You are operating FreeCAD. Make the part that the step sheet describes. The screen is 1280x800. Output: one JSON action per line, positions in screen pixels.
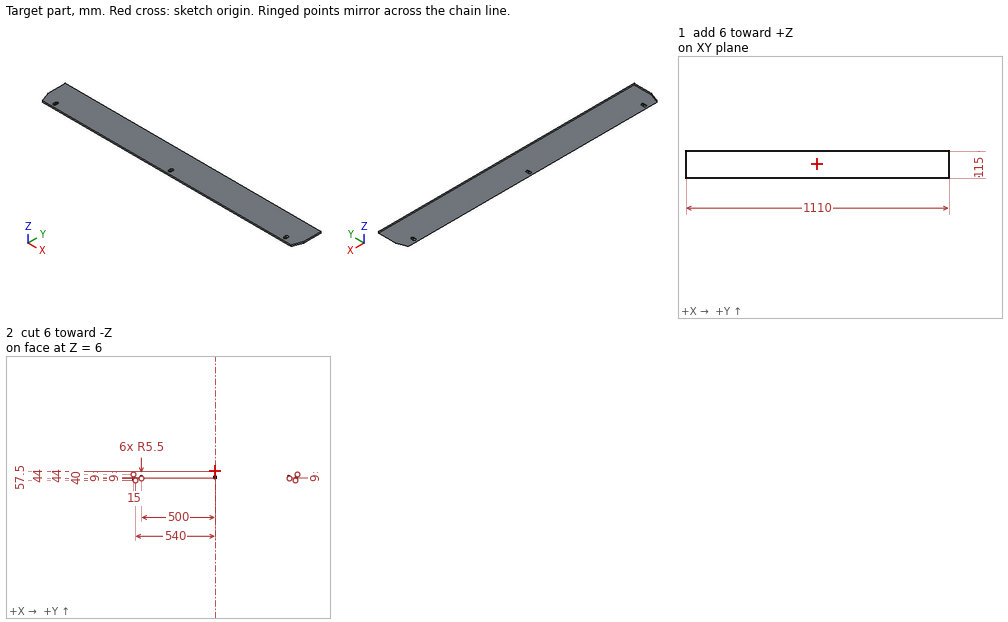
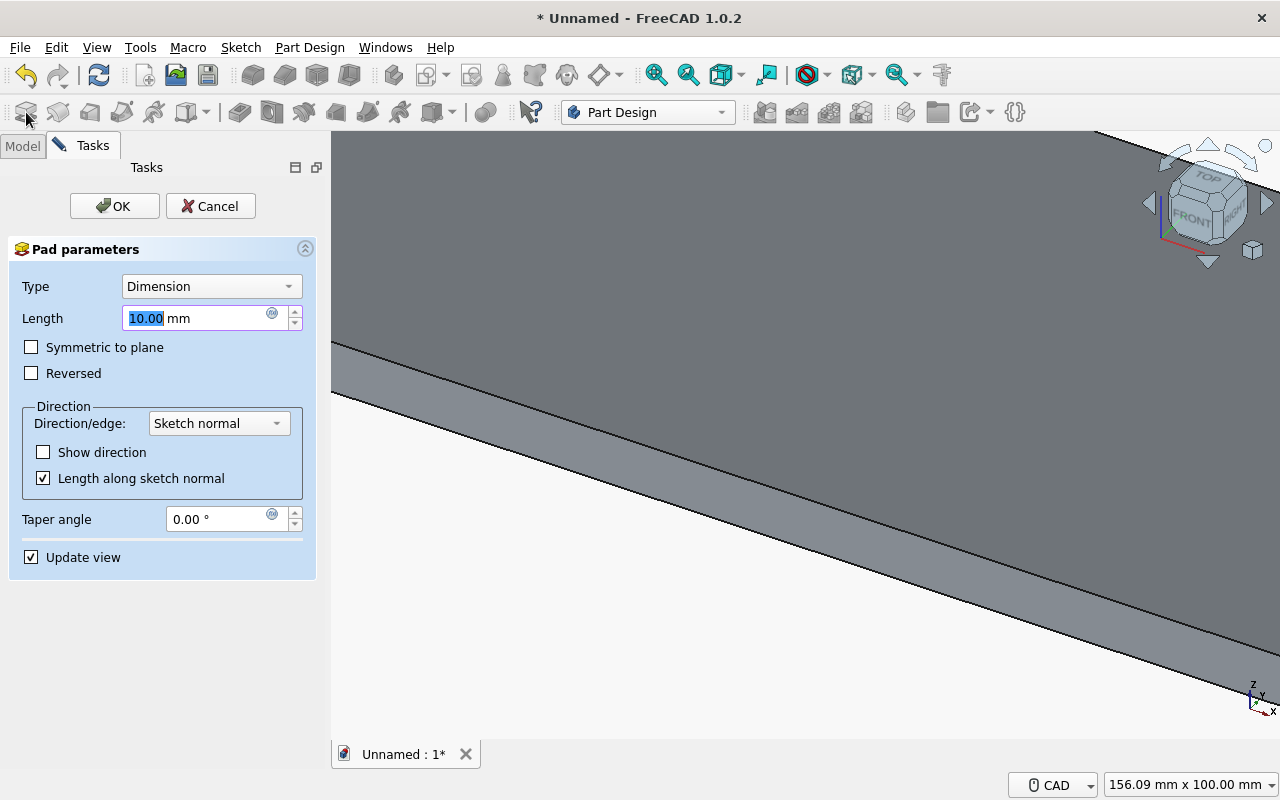
{"action": "type", "text": "6"}
{"action": "key", "text": "Tab"}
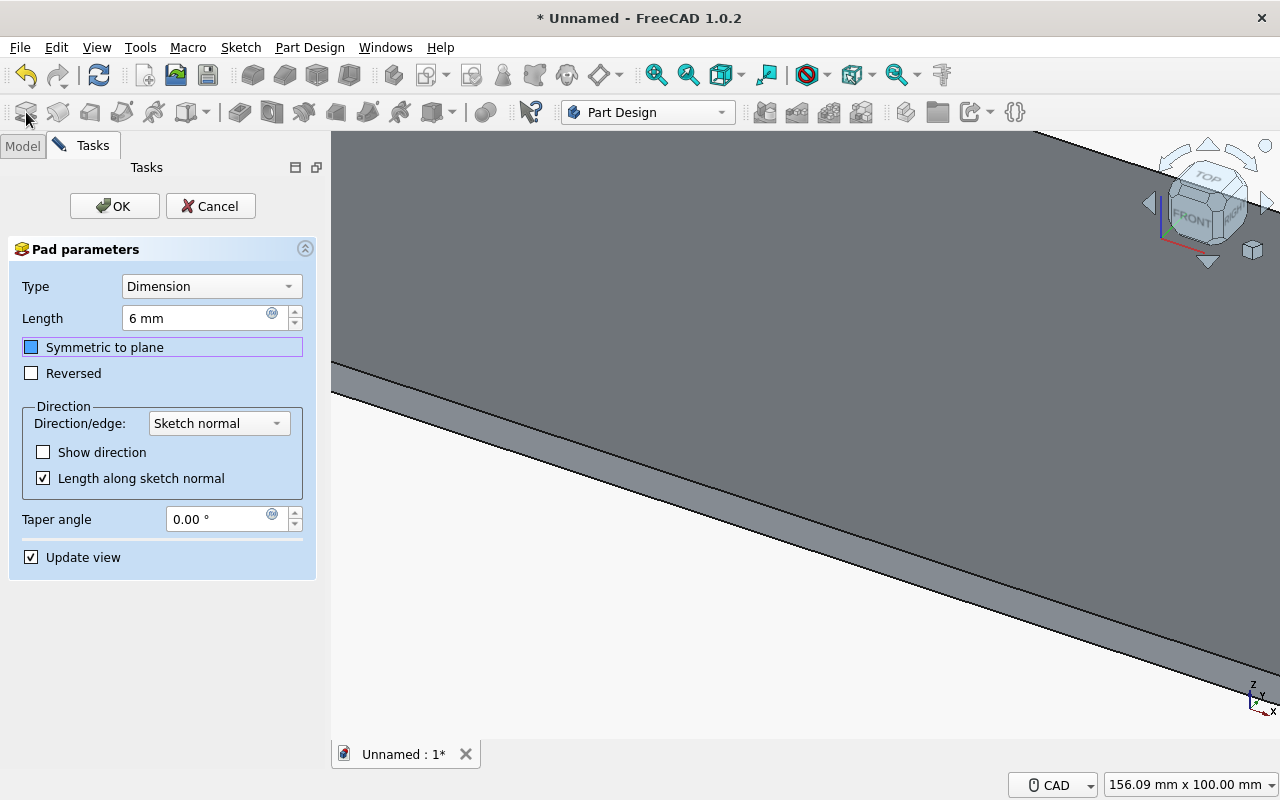
{"action": "left_click", "coordinate": [115, 206]}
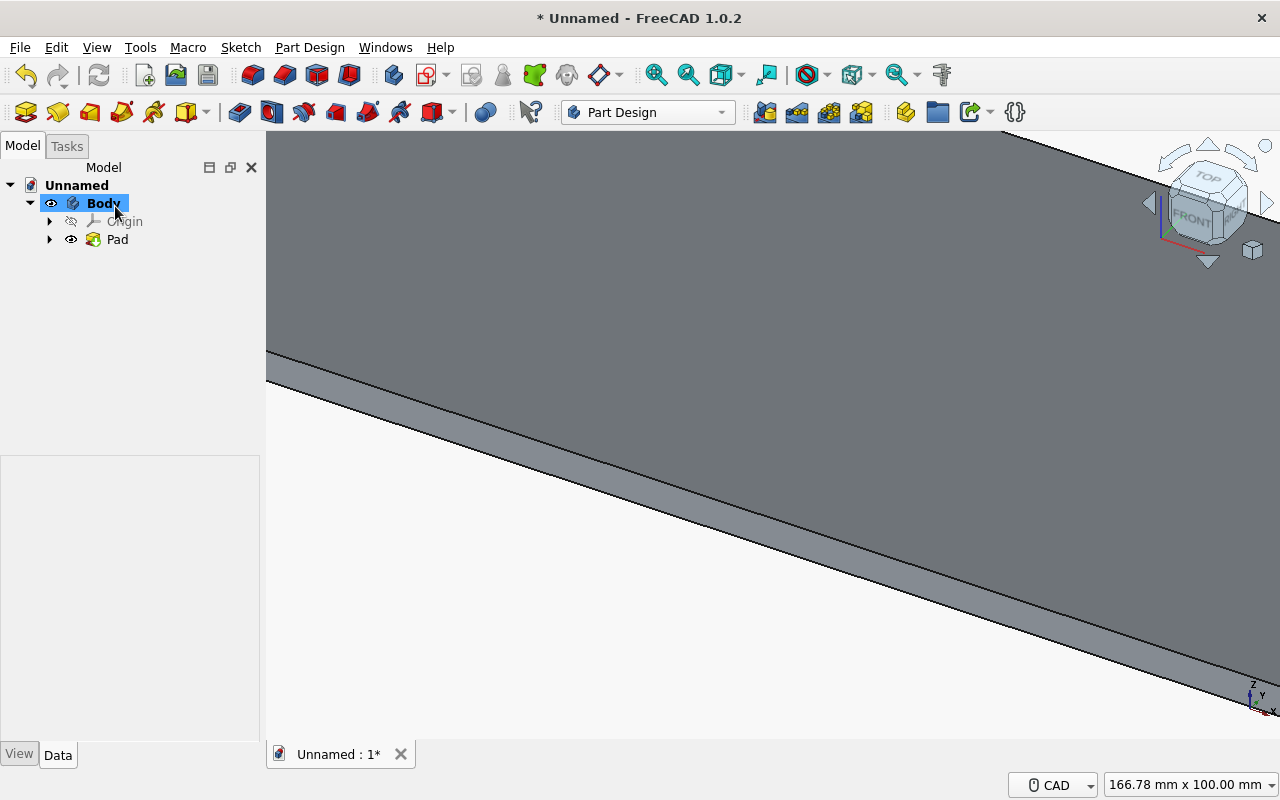
{"action": "left_click", "coordinate": [658, 76]}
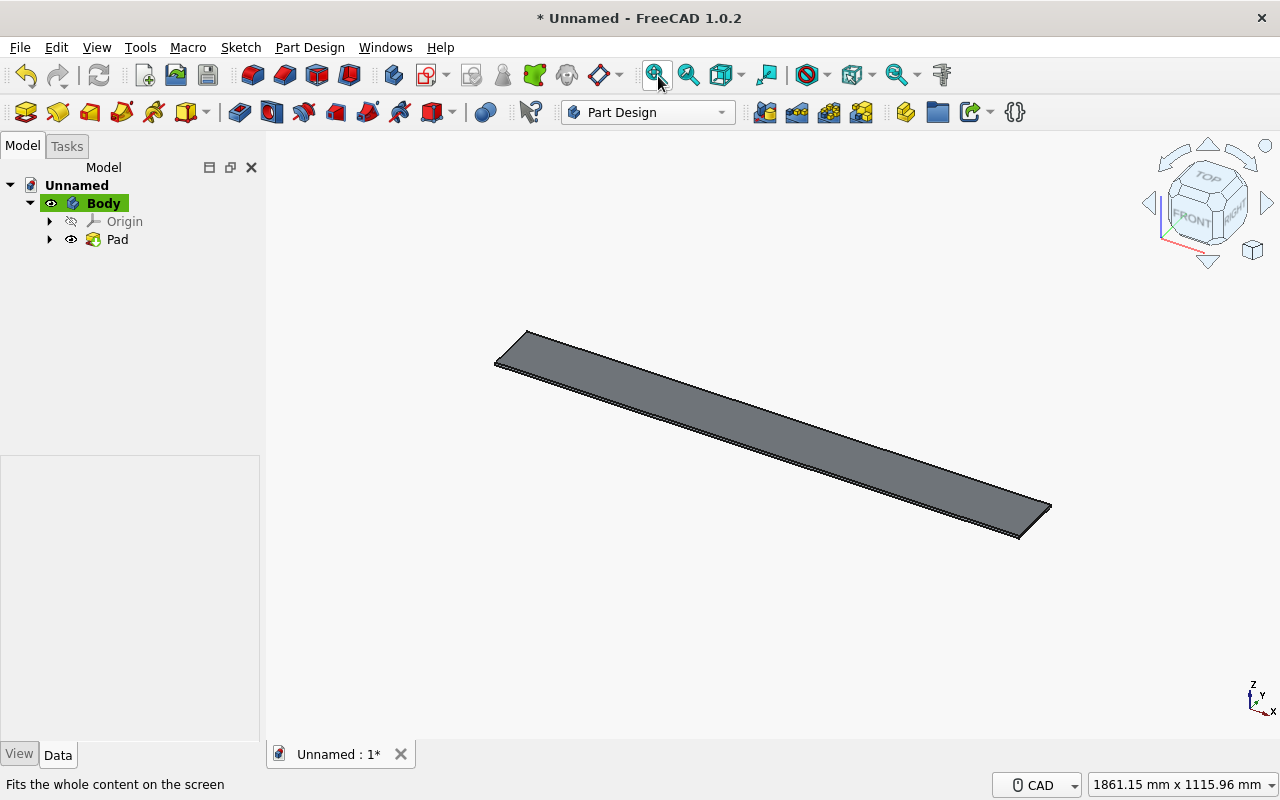
{"action": "left_click", "coordinate": [997, 507]}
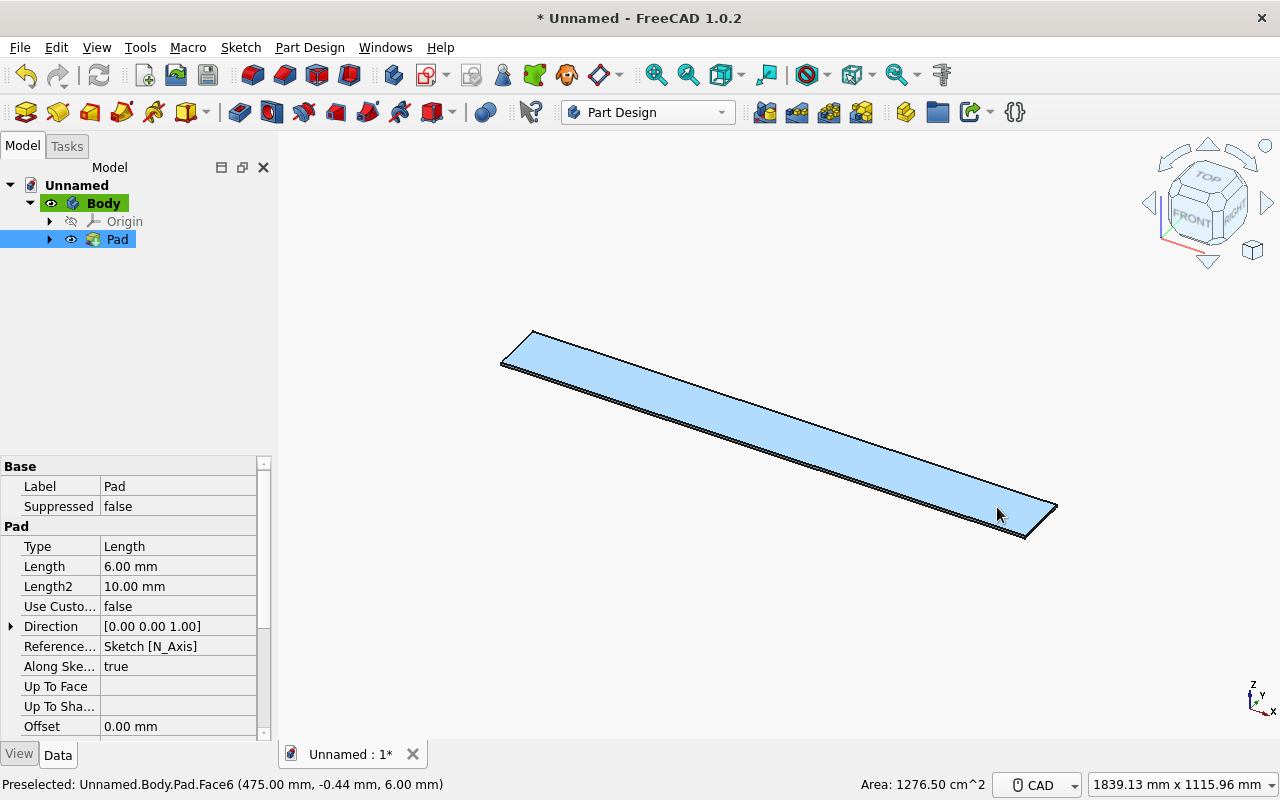
{"action": "left_click", "coordinate": [426, 76]}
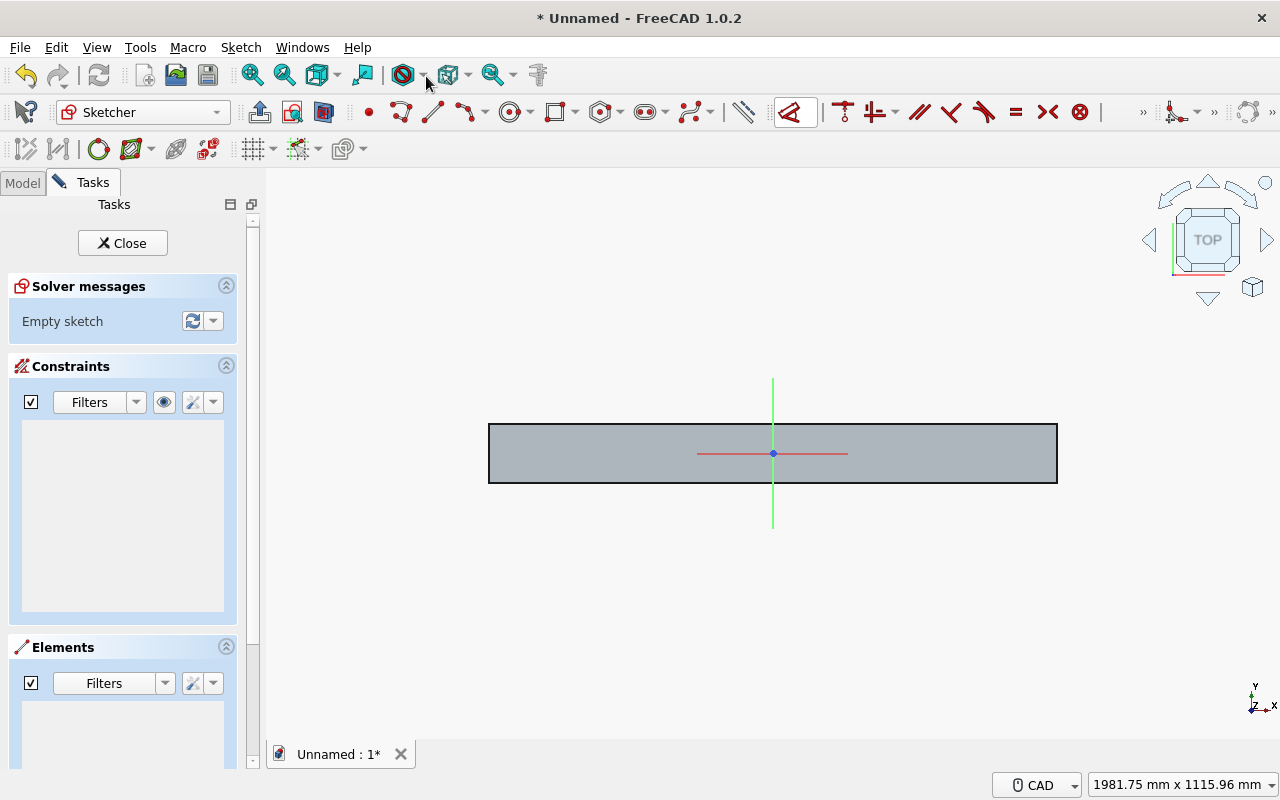
{"action": "left_click", "coordinate": [646, 112]}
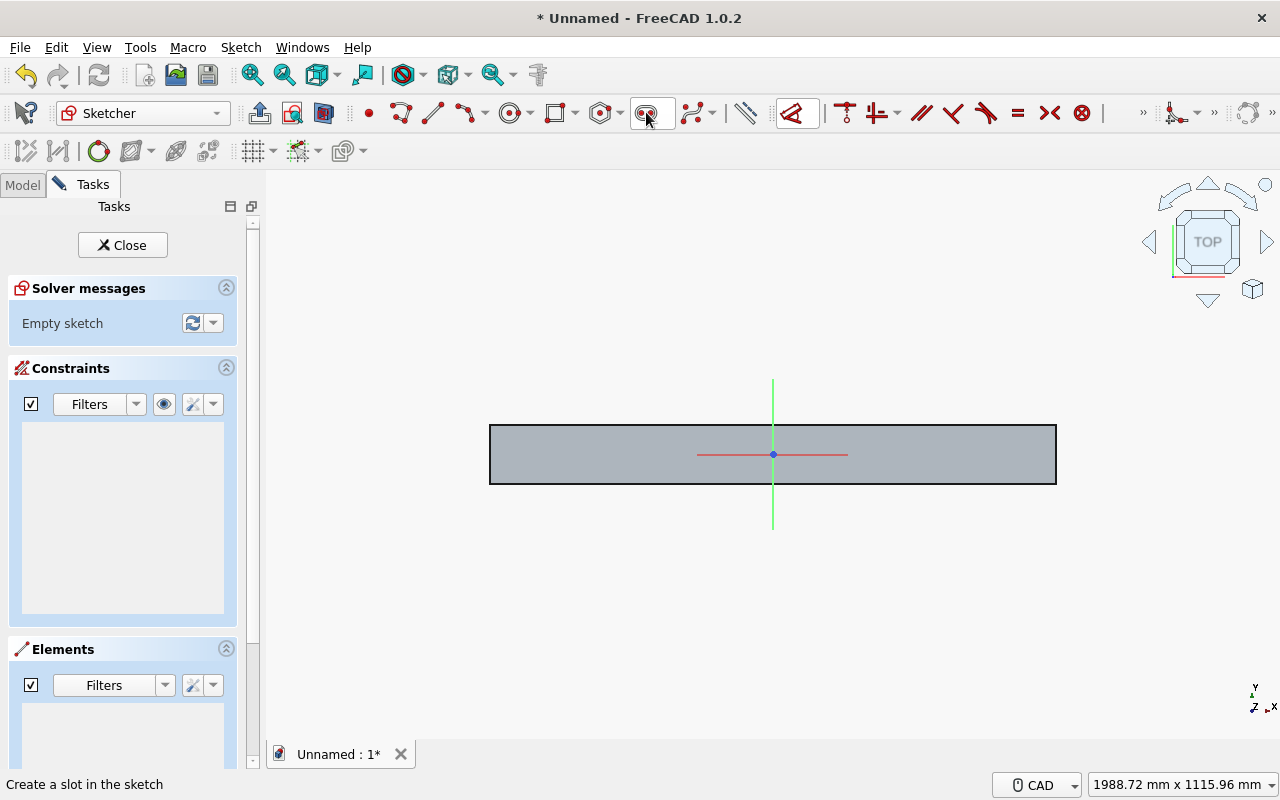
{"action": "scroll", "coordinate": [518, 477], "scroll_direction": "up", "scroll_amount": 11}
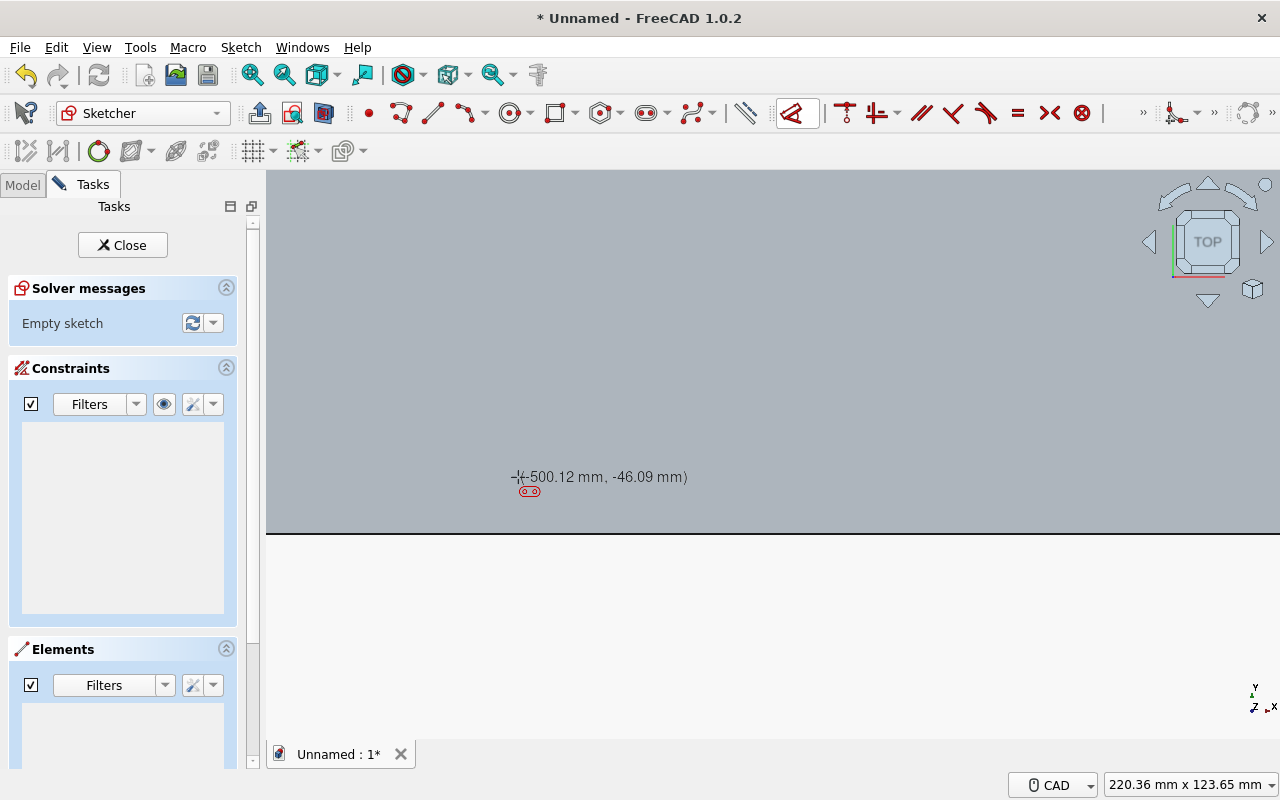
{"action": "scroll", "coordinate": [441, 461], "scroll_direction": "down", "scroll_amount": 11}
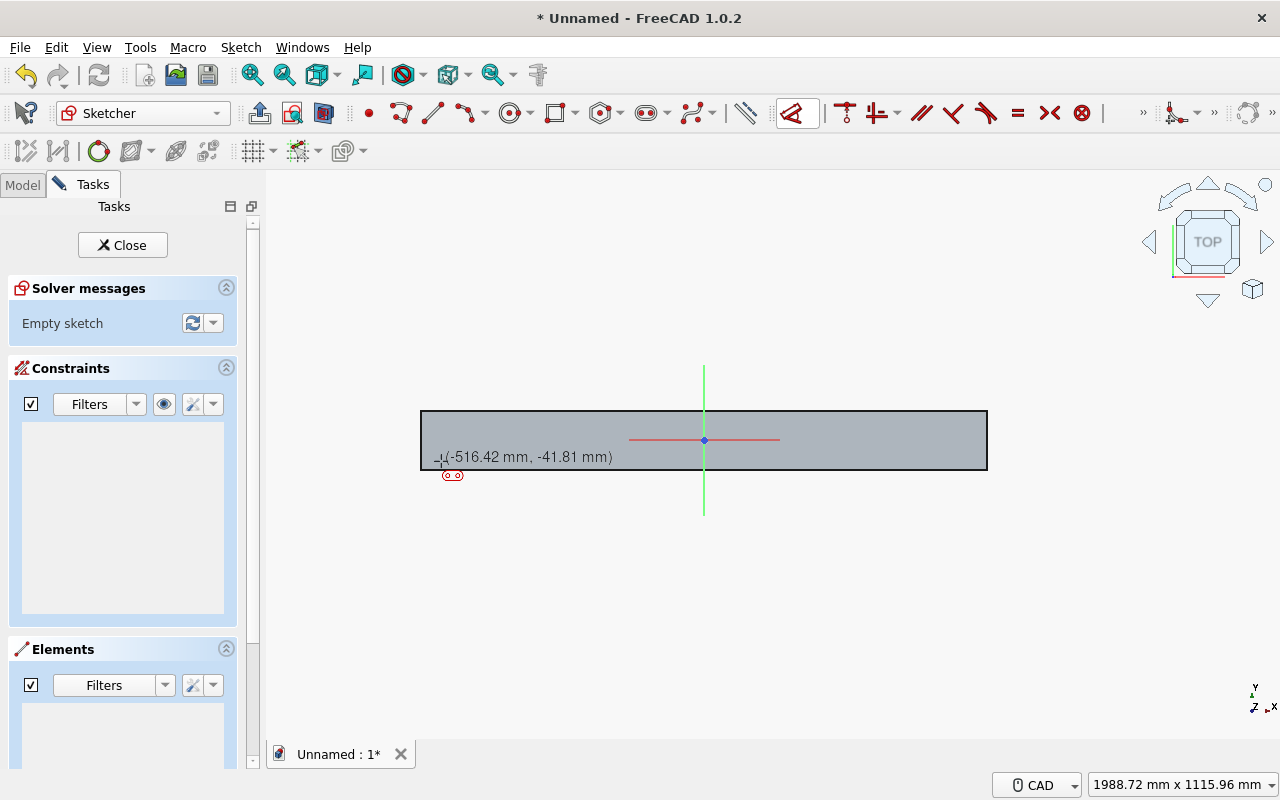
{"action": "left_click", "coordinate": [450, 463]}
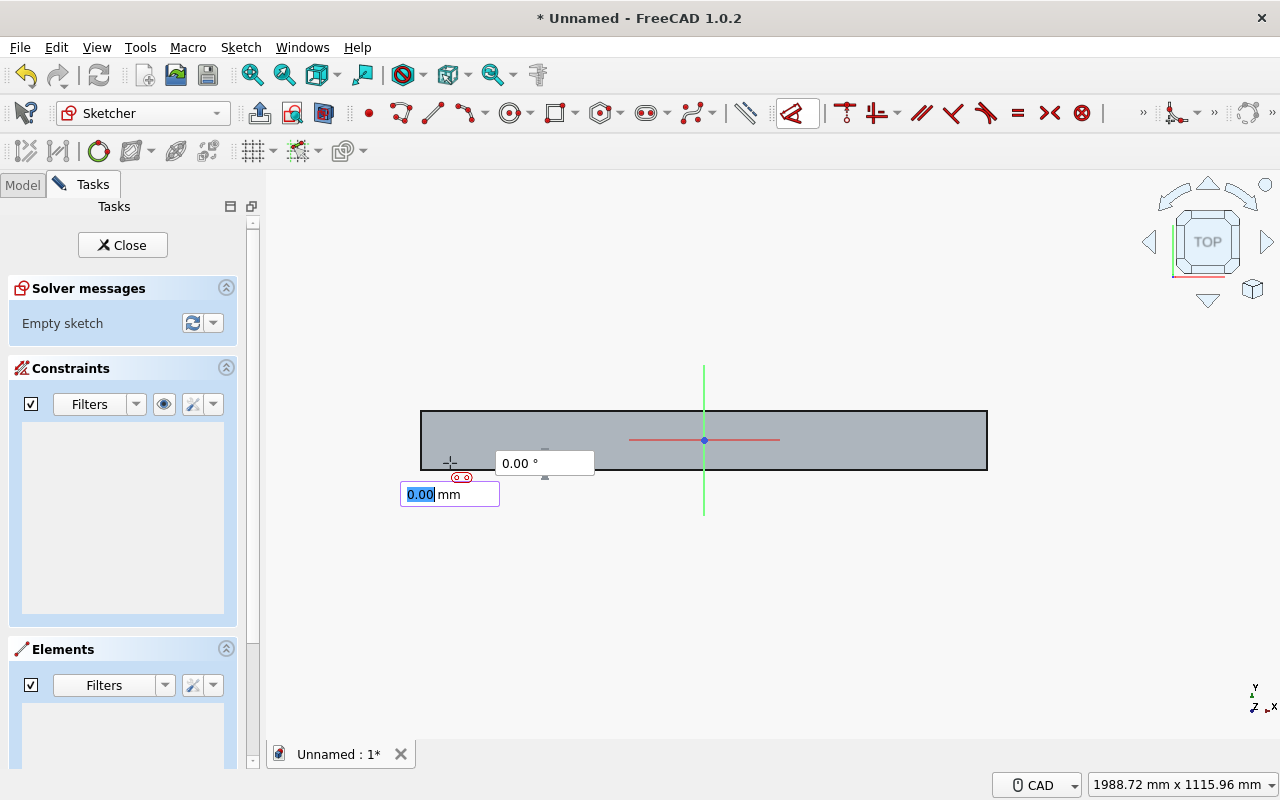
{"action": "scroll", "coordinate": [450, 458], "scroll_direction": "up", "scroll_amount": 7}